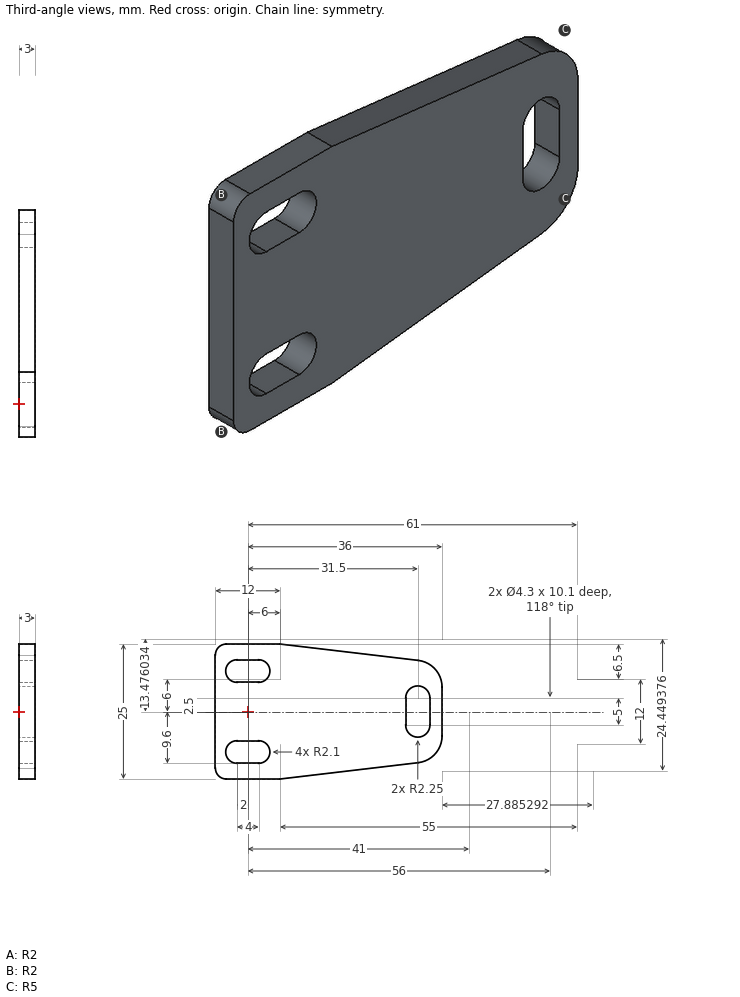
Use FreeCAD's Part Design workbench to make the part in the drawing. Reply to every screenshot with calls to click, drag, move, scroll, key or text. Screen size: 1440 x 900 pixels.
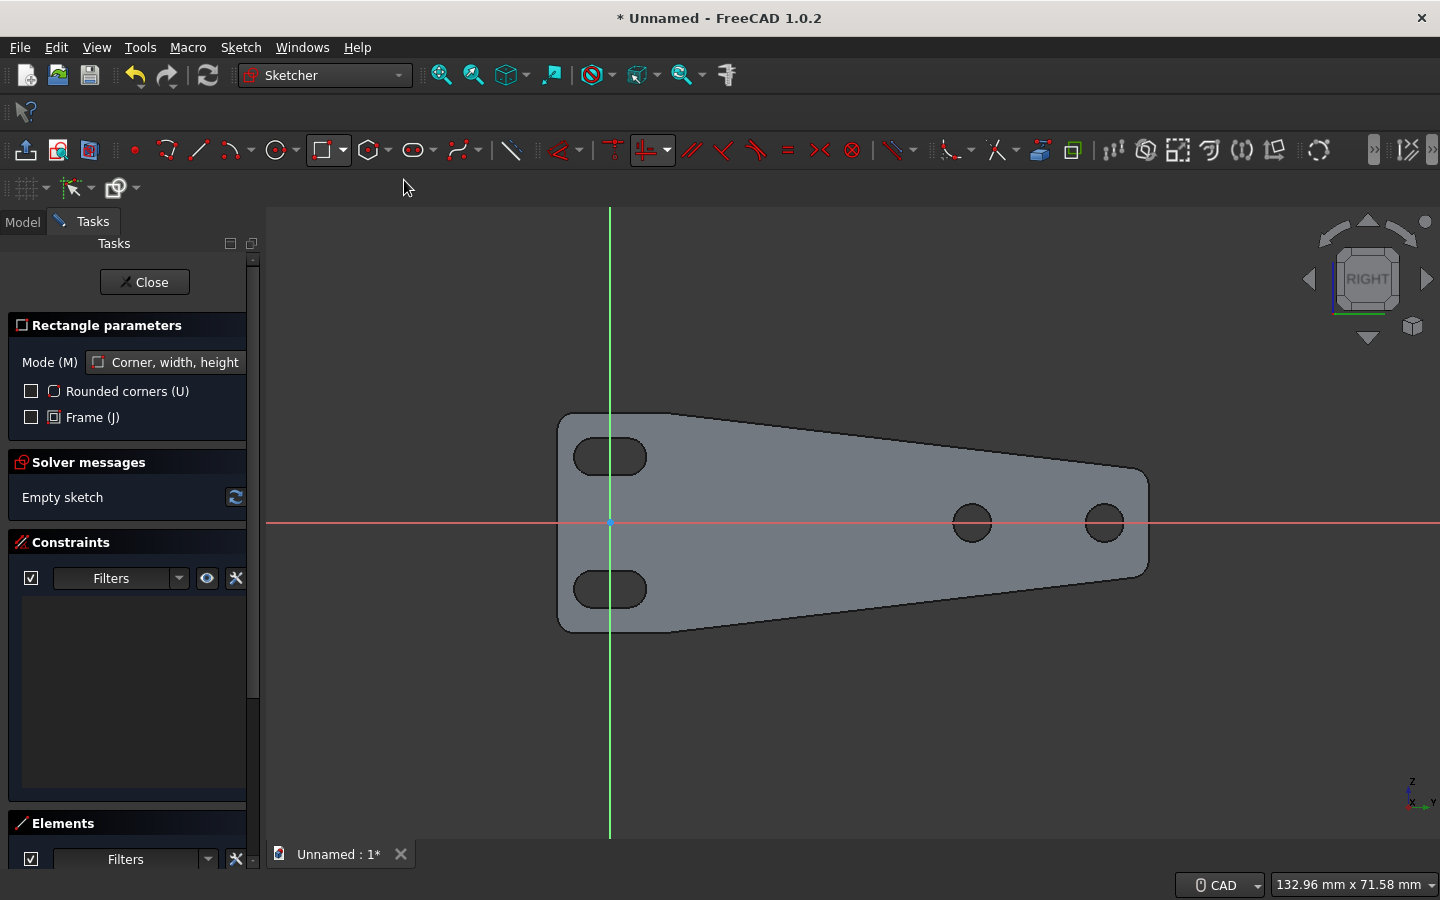
click(928, 404)
click(1174, 620)
key(Escape)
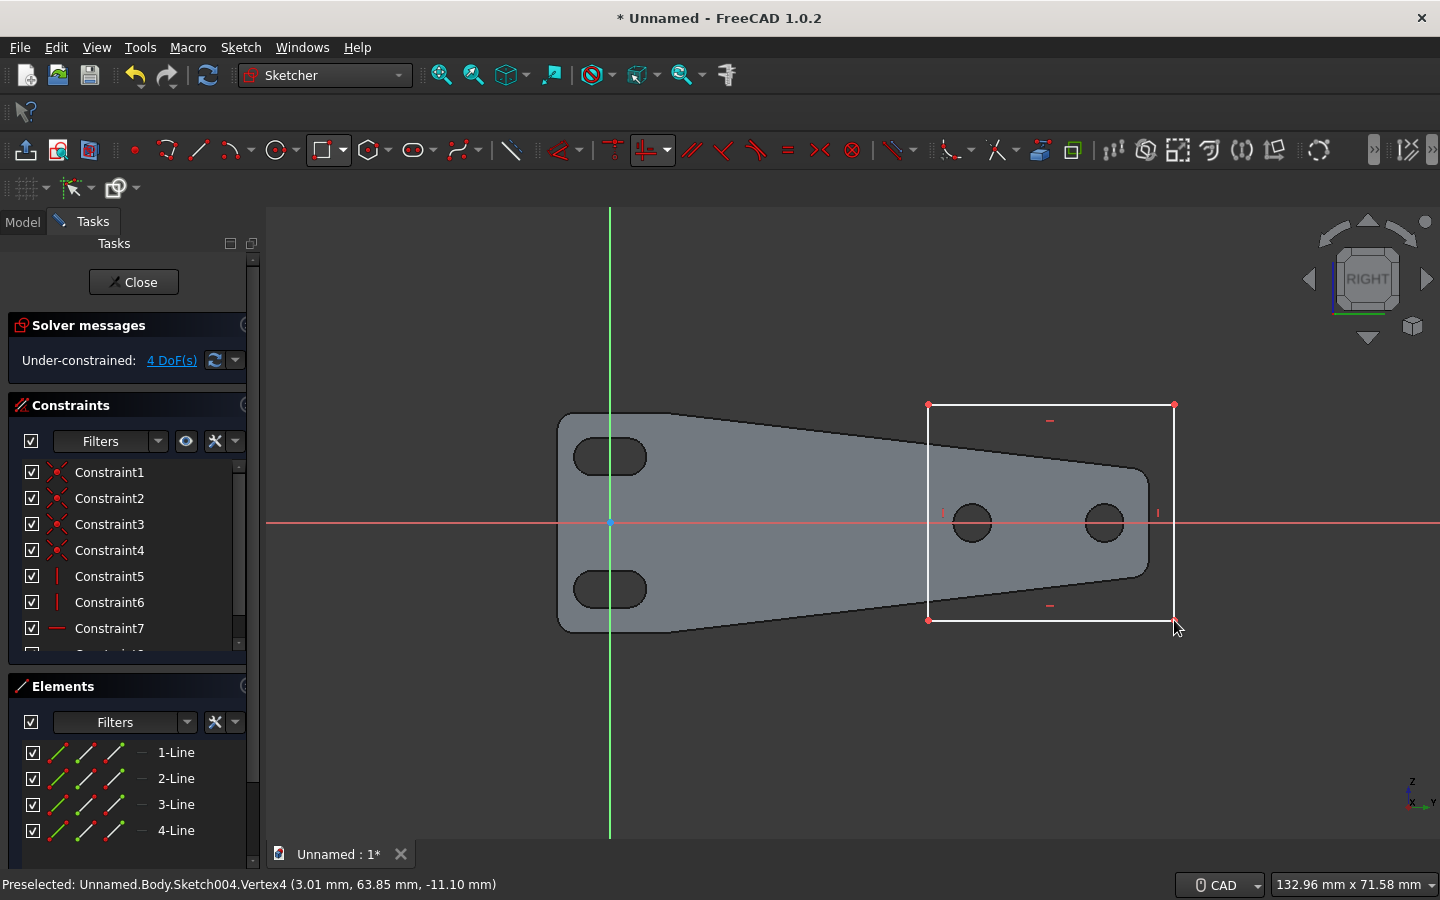
click(558, 150)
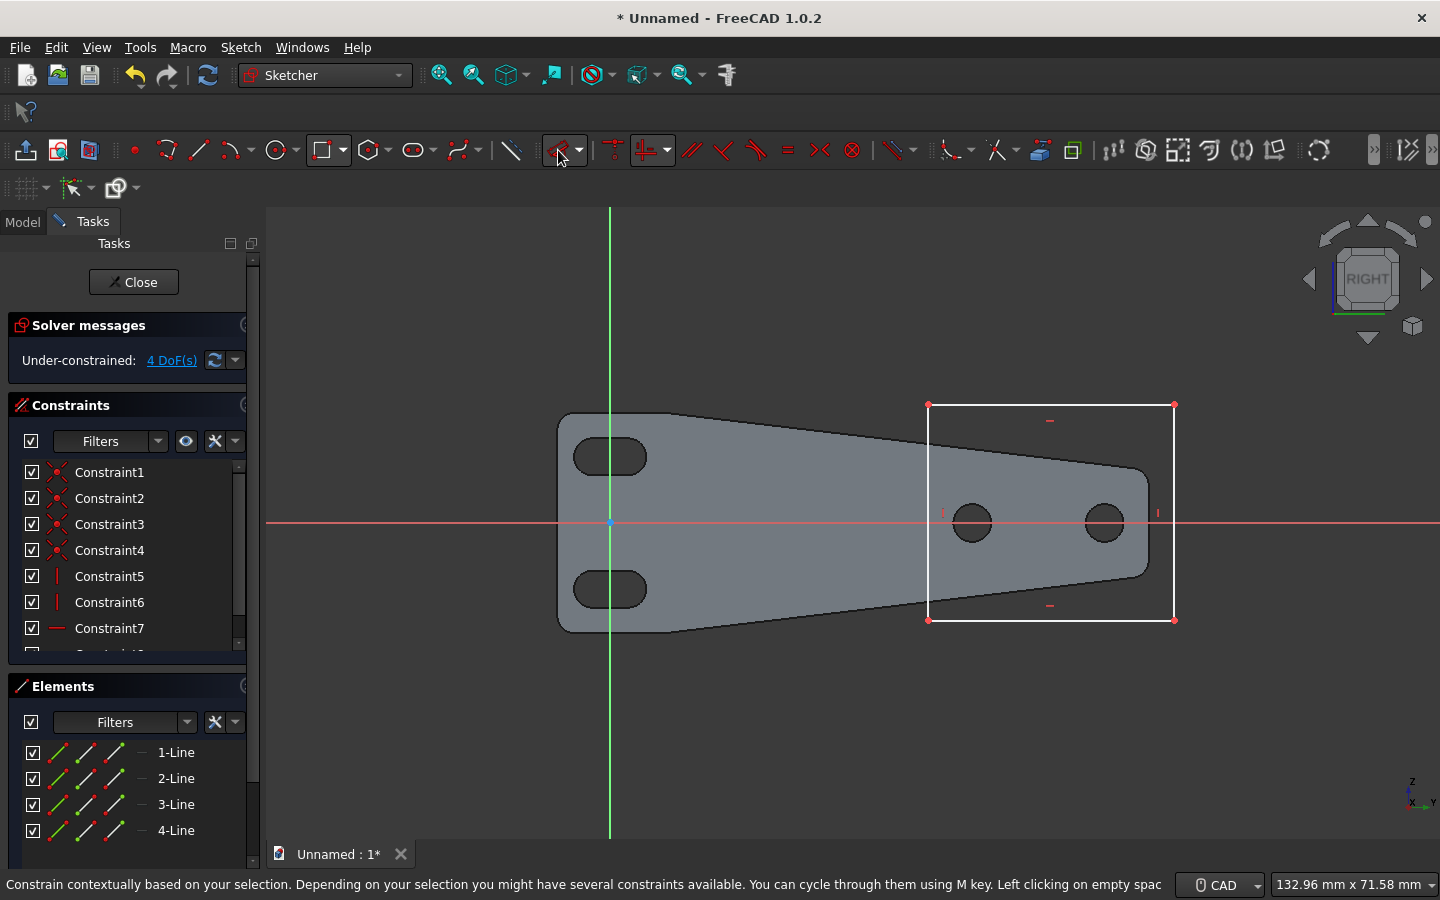
click(928, 405)
click(769, 371)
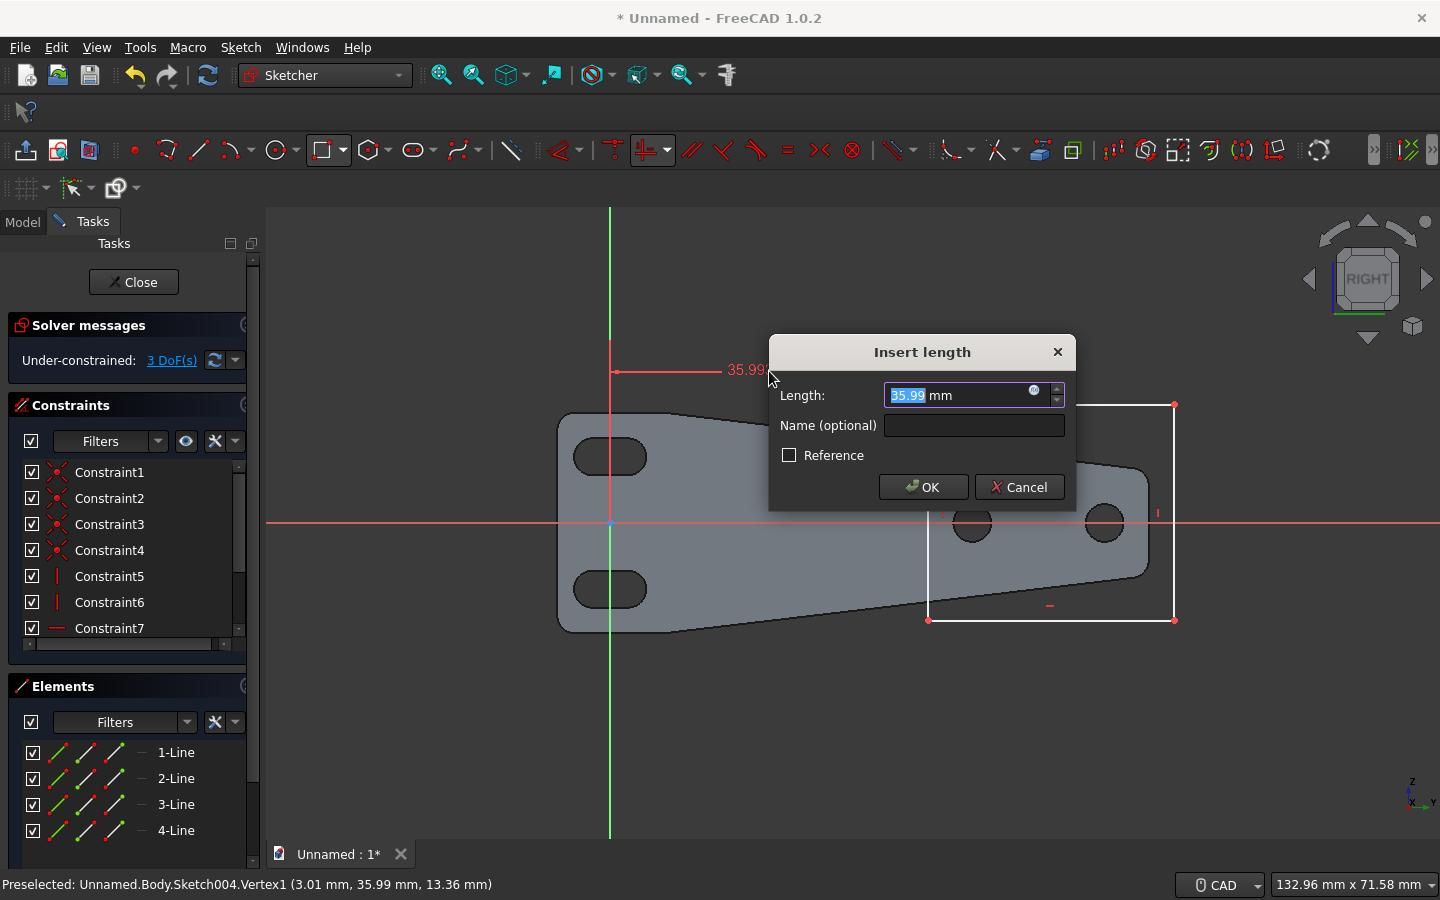
text(36)
key(Return)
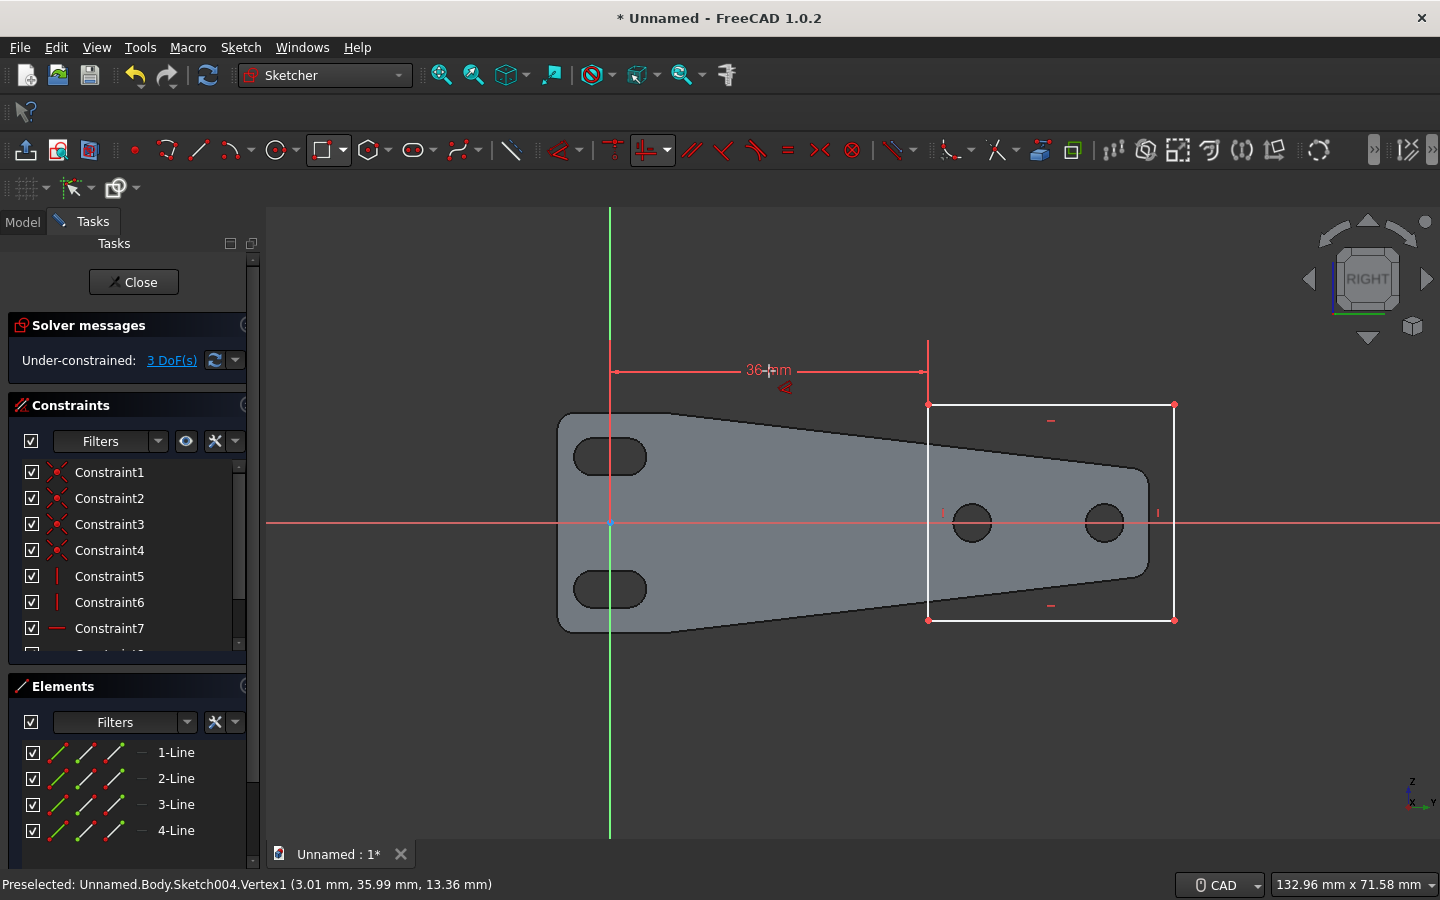
click(928, 470)
click(962, 463)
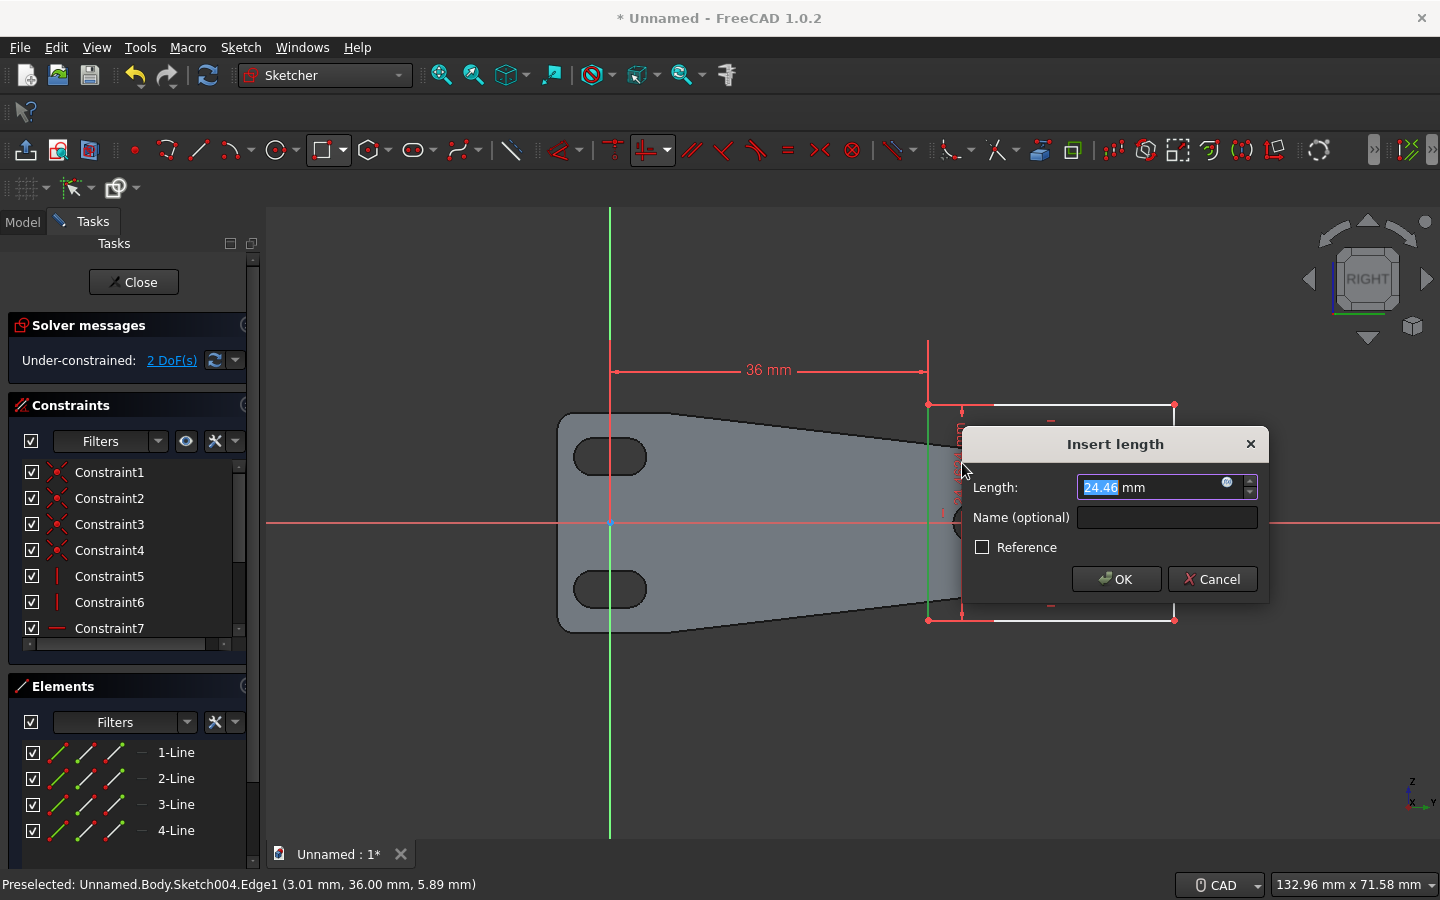
text(24.449376)
key(Return)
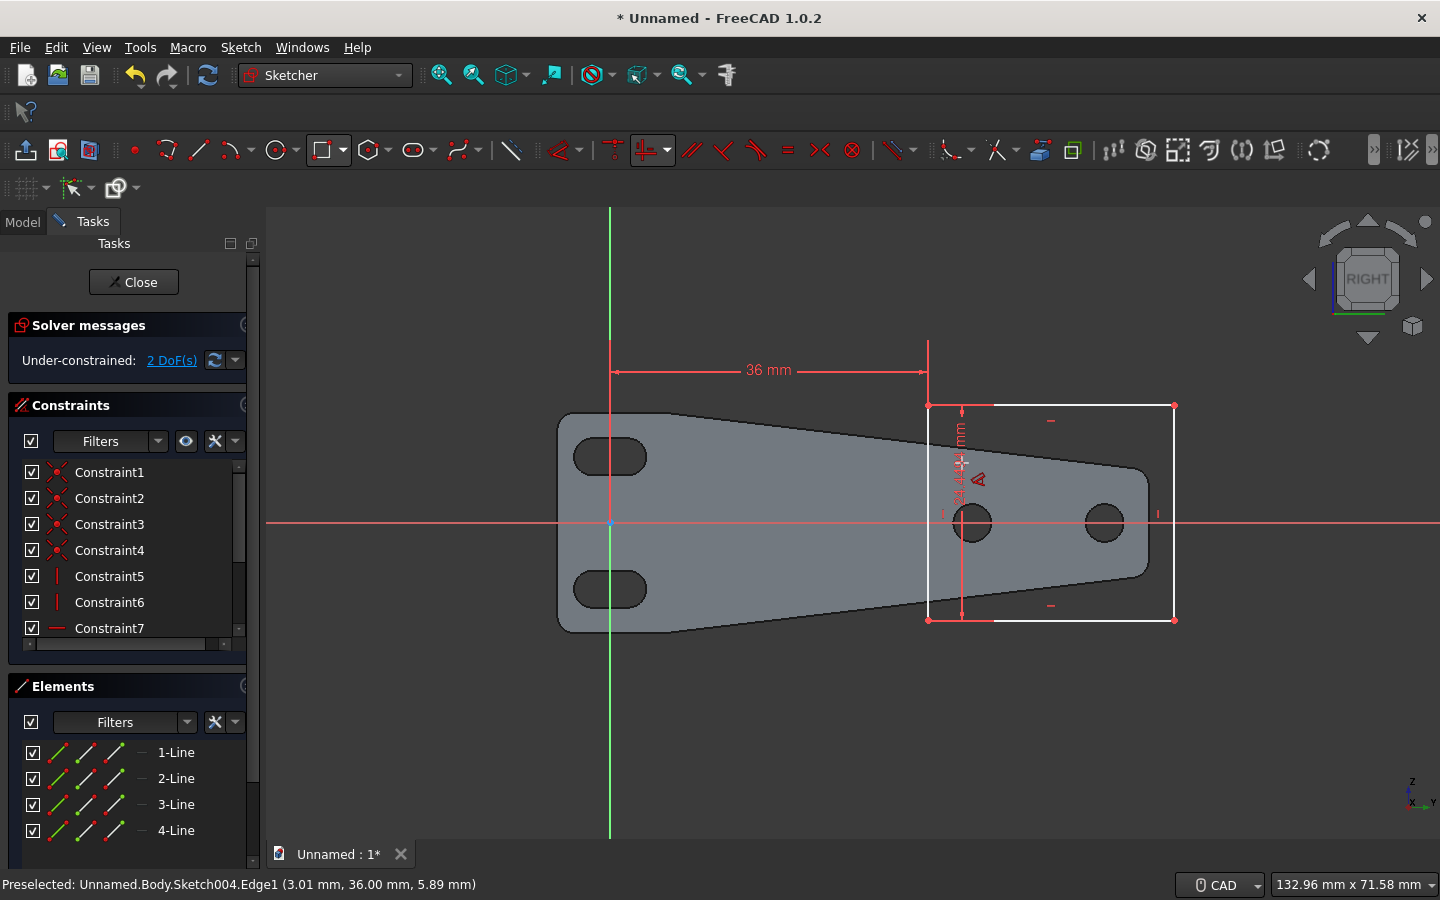
click(1002, 621)
click(1051, 655)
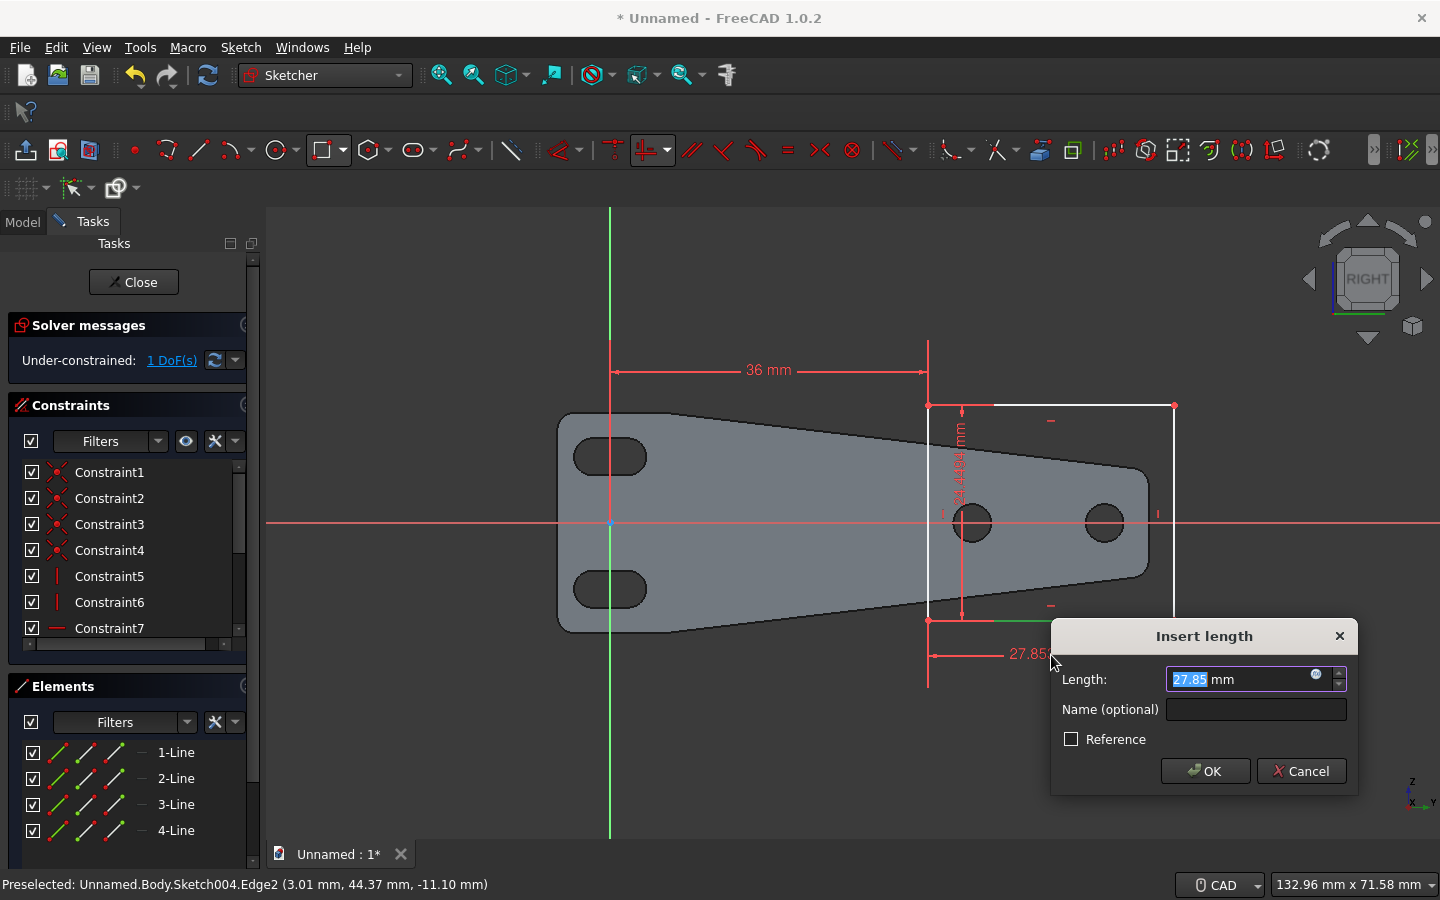
text(27.885292)
key(Return)